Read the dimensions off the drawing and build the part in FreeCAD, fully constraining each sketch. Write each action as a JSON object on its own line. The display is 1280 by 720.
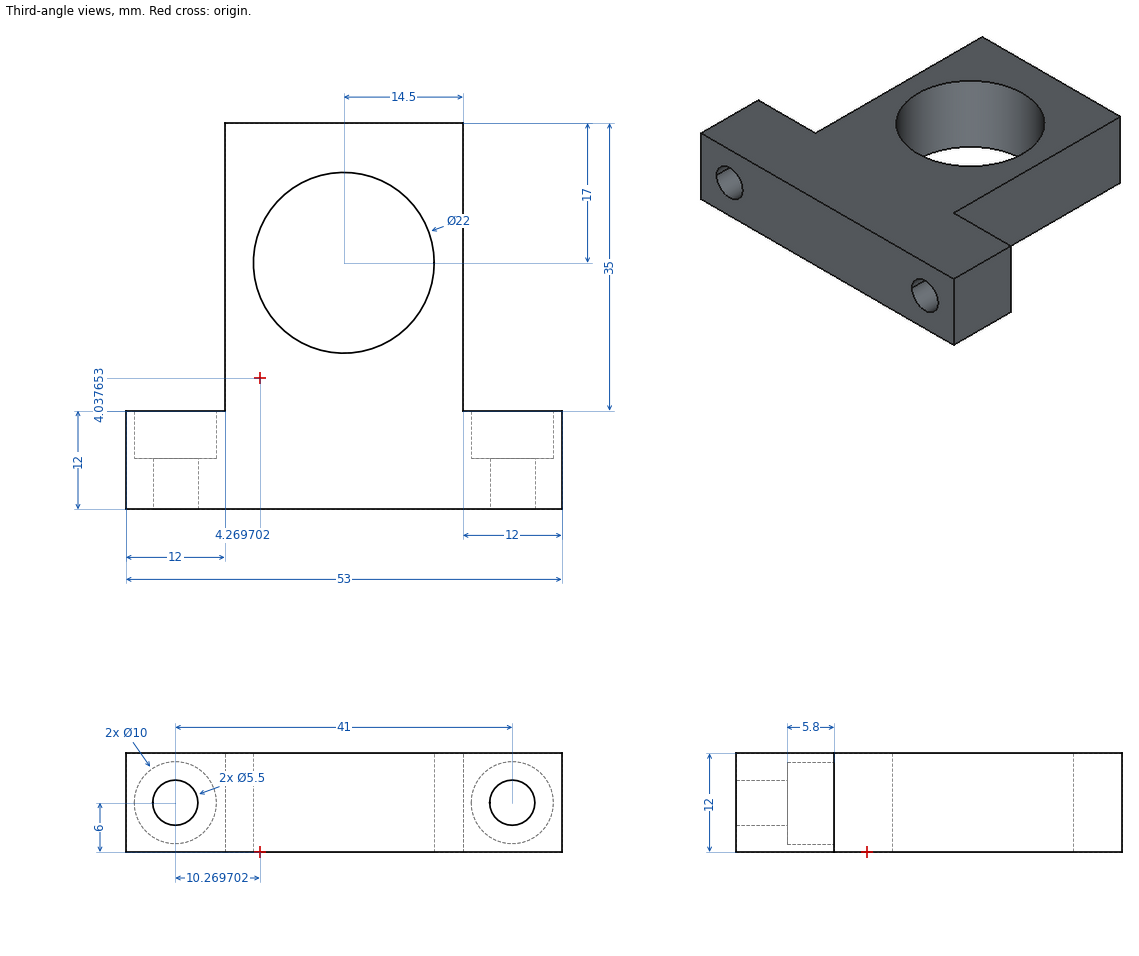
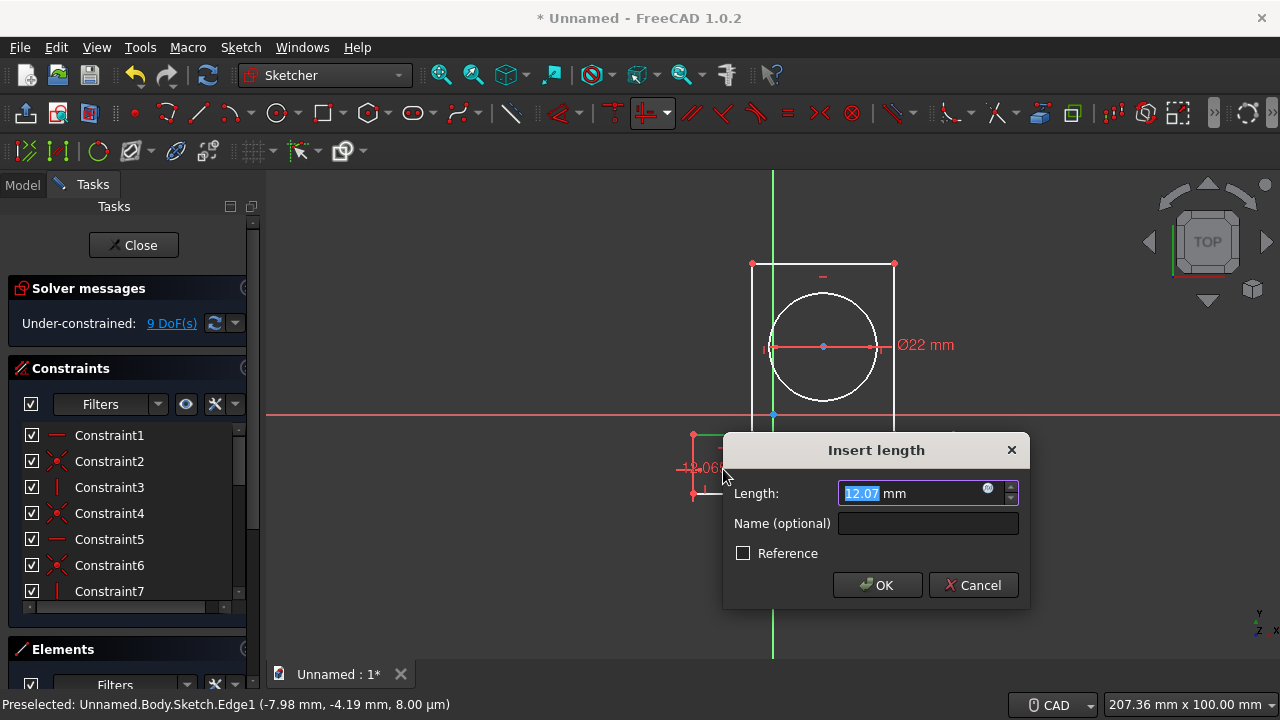
{"action": "type", "text": "12"}
{"action": "key", "text": "Return"}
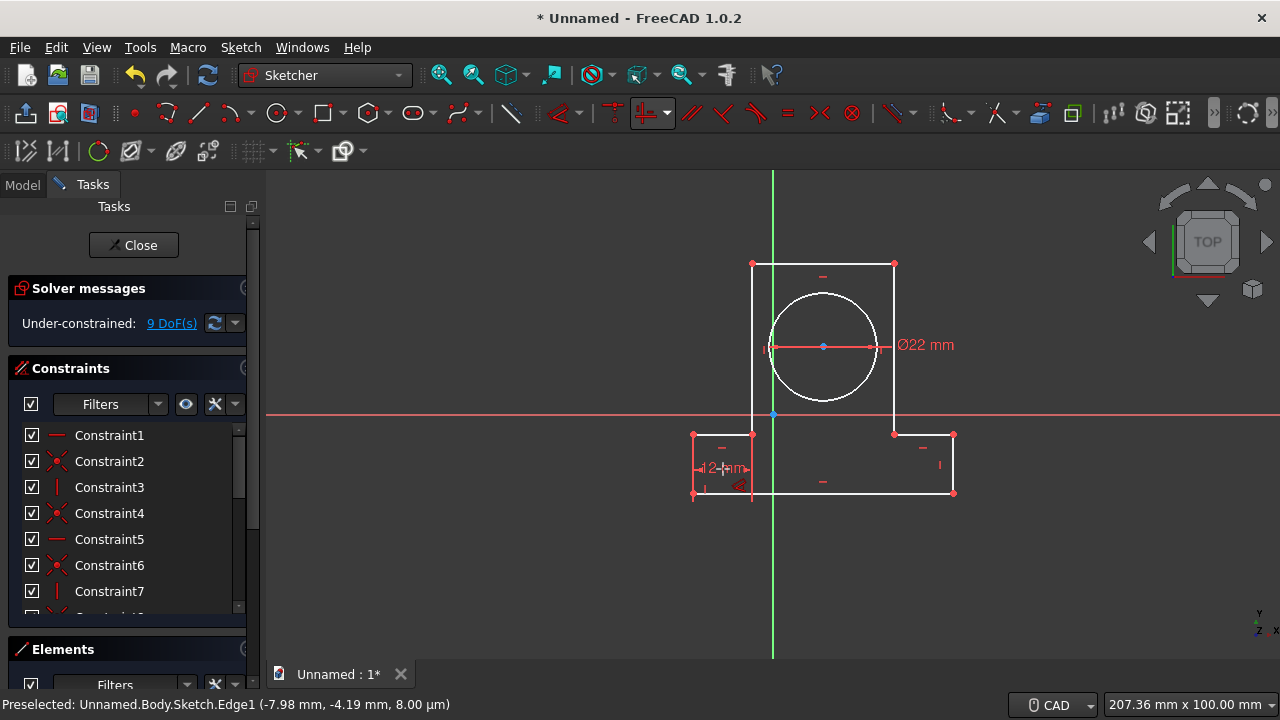
{"action": "left_click", "coordinate": [693, 453]}
{"action": "left_click", "coordinate": [659, 444]}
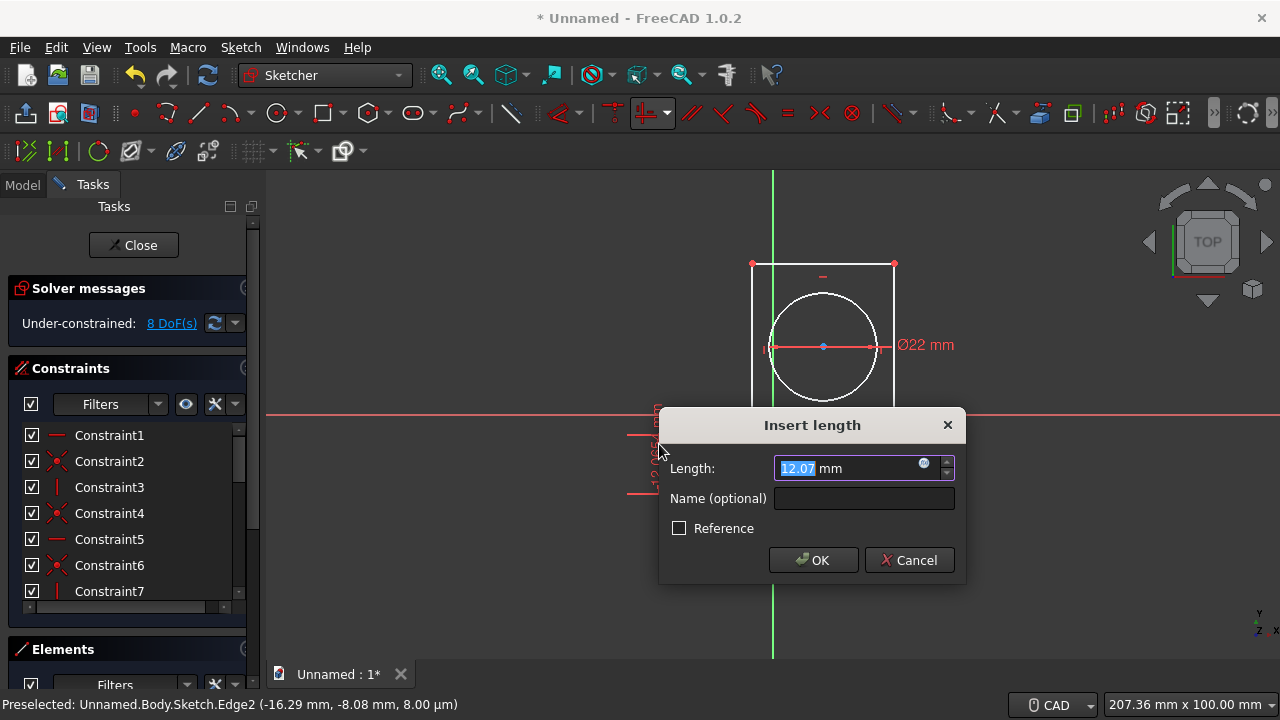
{"action": "type", "text": "12"}
{"action": "key", "text": "Return"}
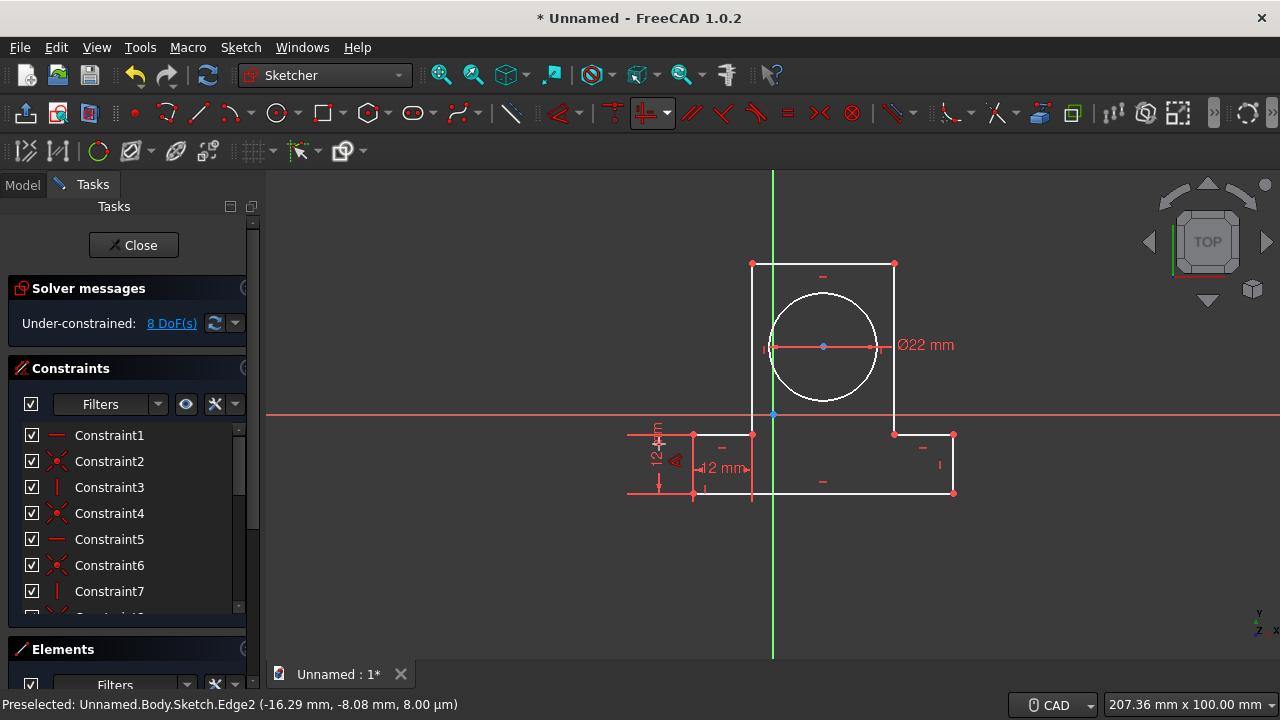
{"action": "left_click", "coordinate": [771, 494]}
{"action": "left_click", "coordinate": [823, 528]}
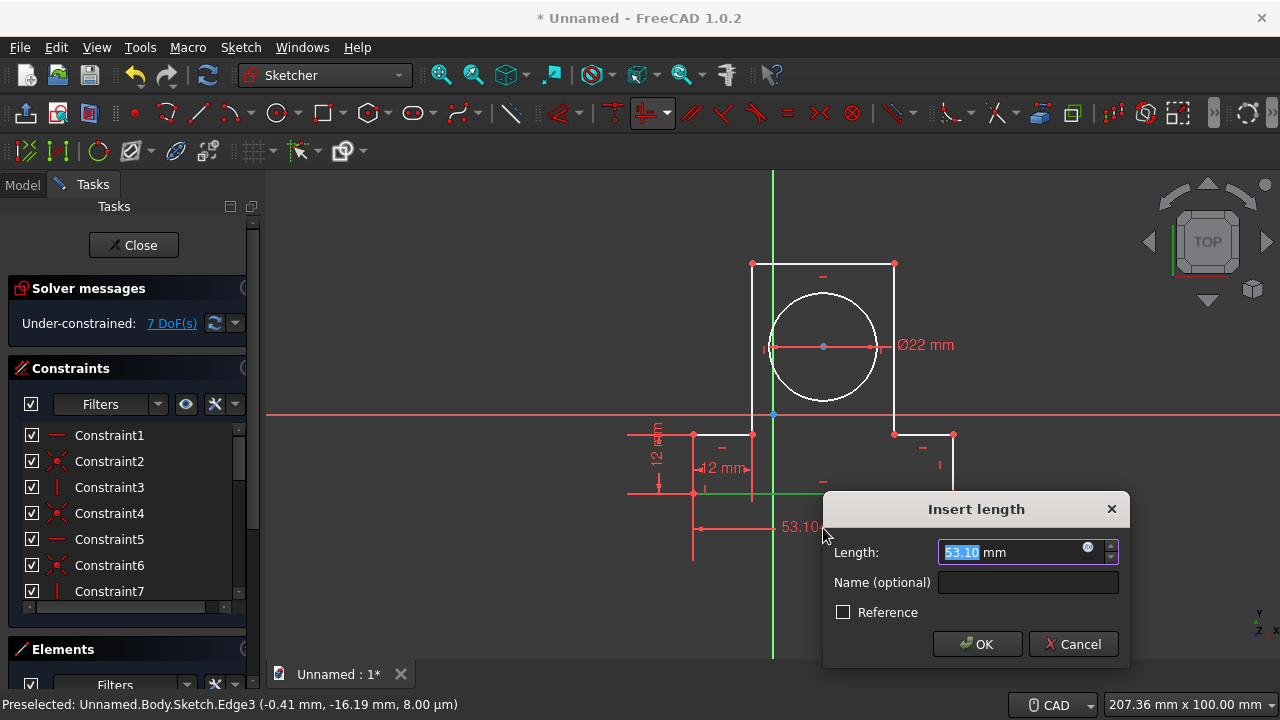
{"action": "type", "text": "53"}
{"action": "key", "text": "Return"}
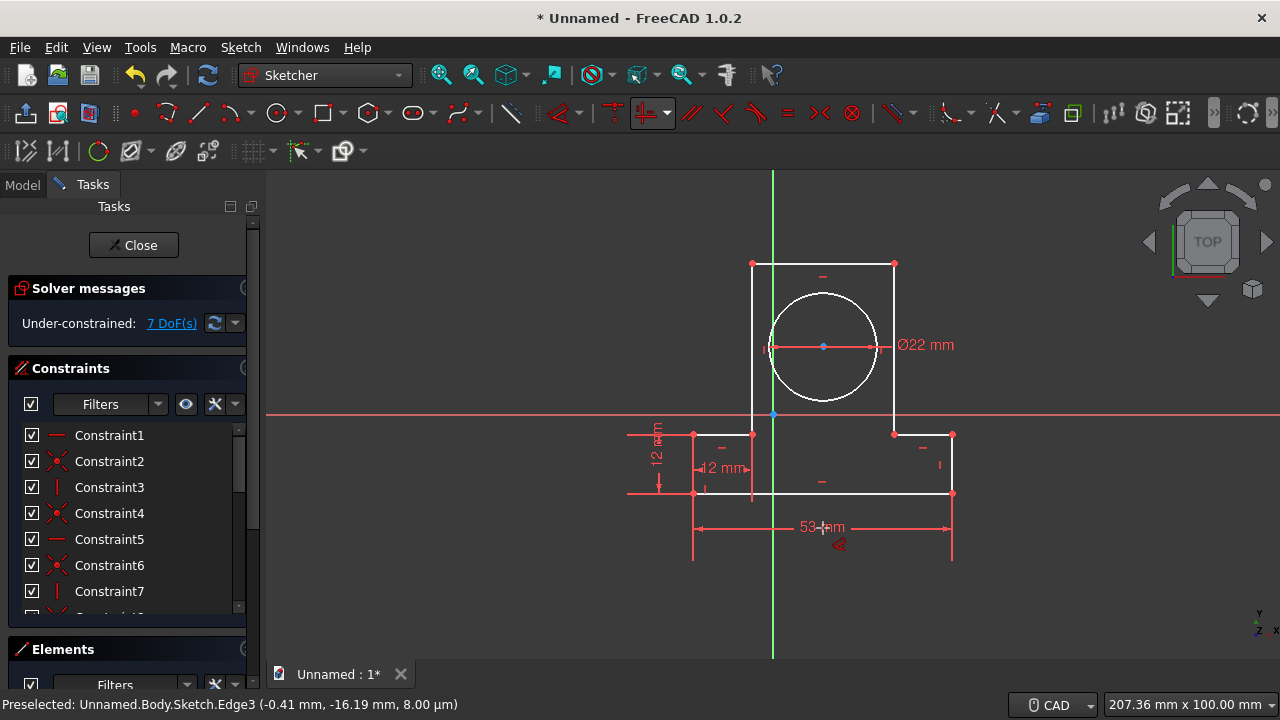
{"action": "left_click", "coordinate": [952, 476]}
{"action": "left_click", "coordinate": [986, 464]}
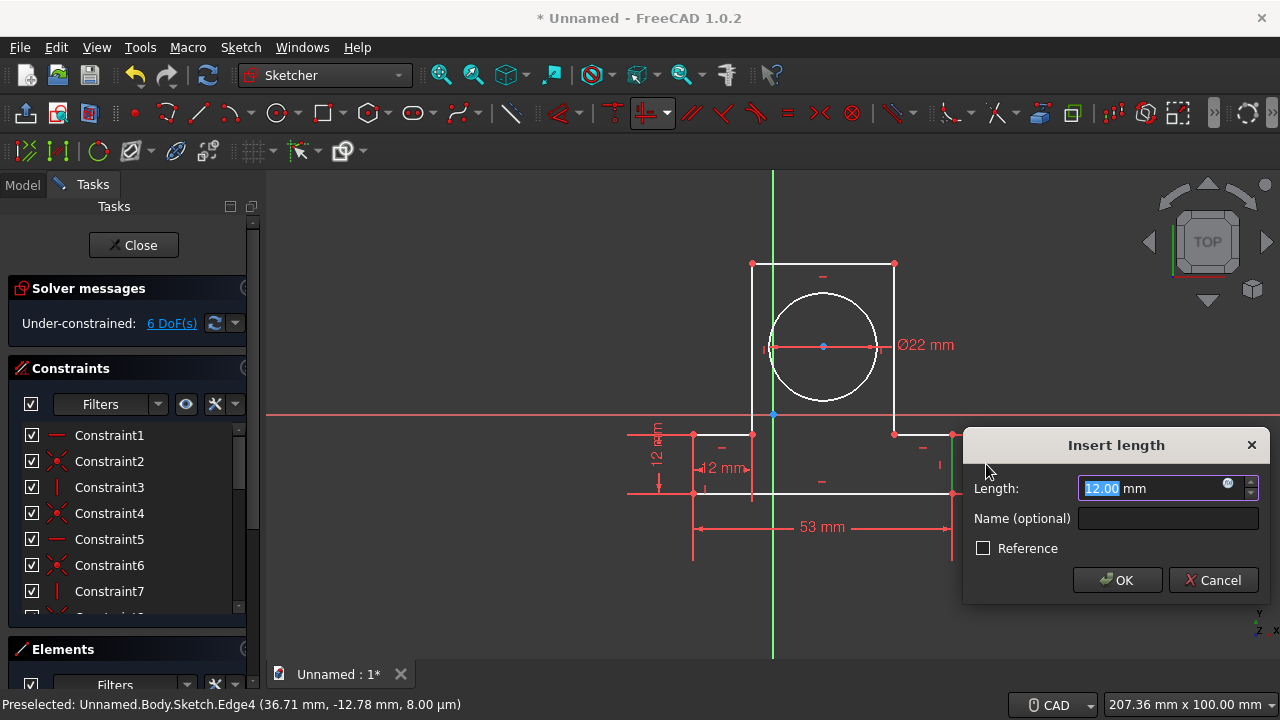
{"action": "type", "text": "12"}
{"action": "key", "text": "Return"}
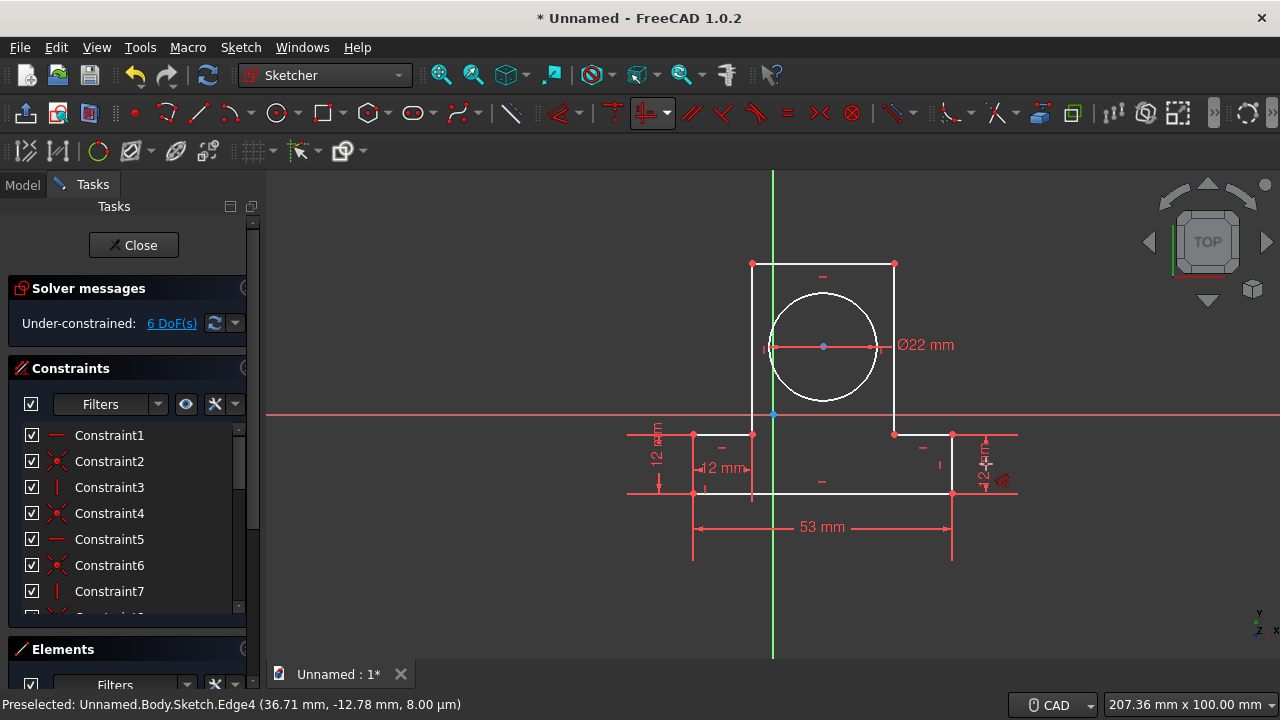
{"action": "left_click", "coordinate": [935, 435]}
{"action": "left_click", "coordinate": [910, 469]}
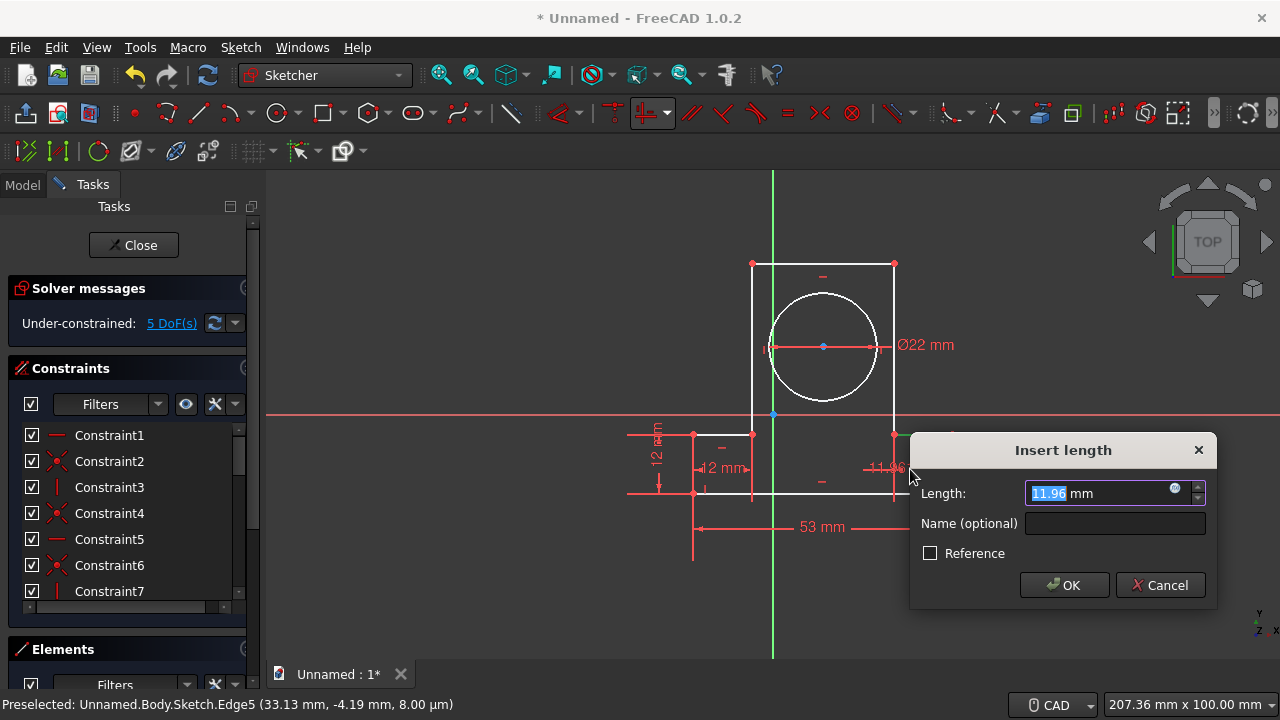
{"action": "type", "text": "12"}
{"action": "key", "text": "Return"}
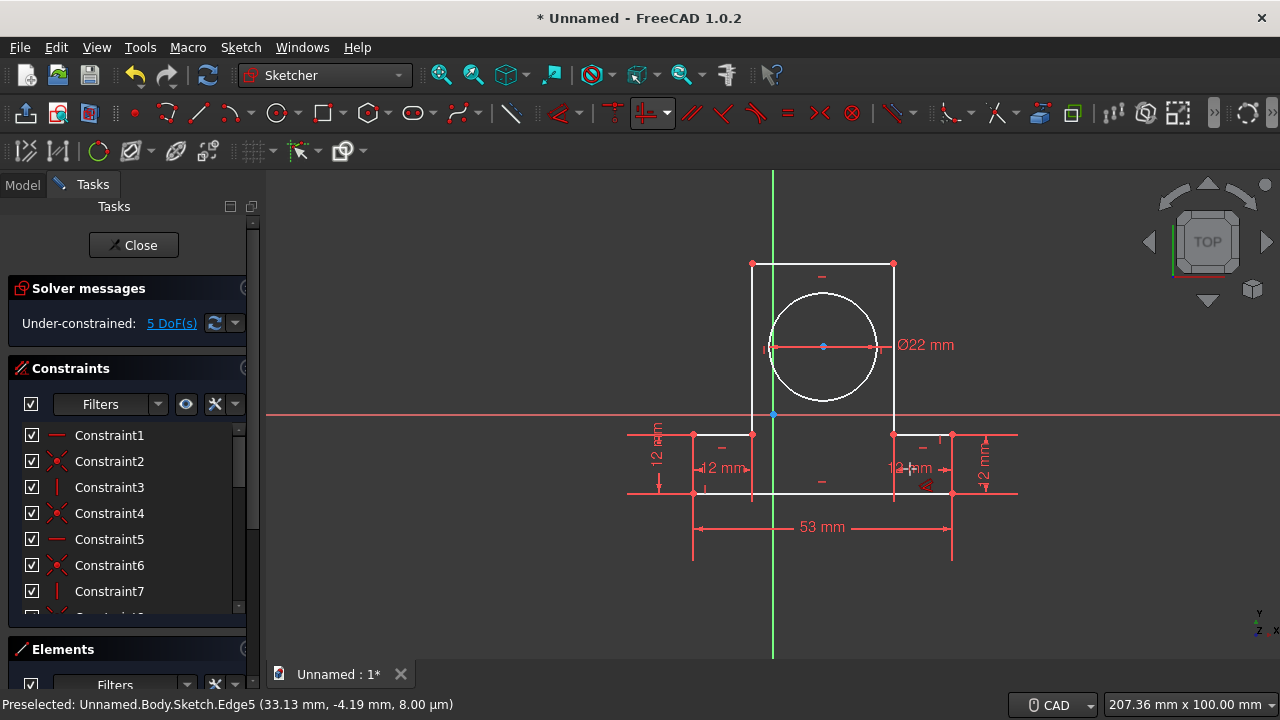
{"action": "left_click", "coordinate": [894, 384]}
{"action": "left_click", "coordinate": [928, 350]}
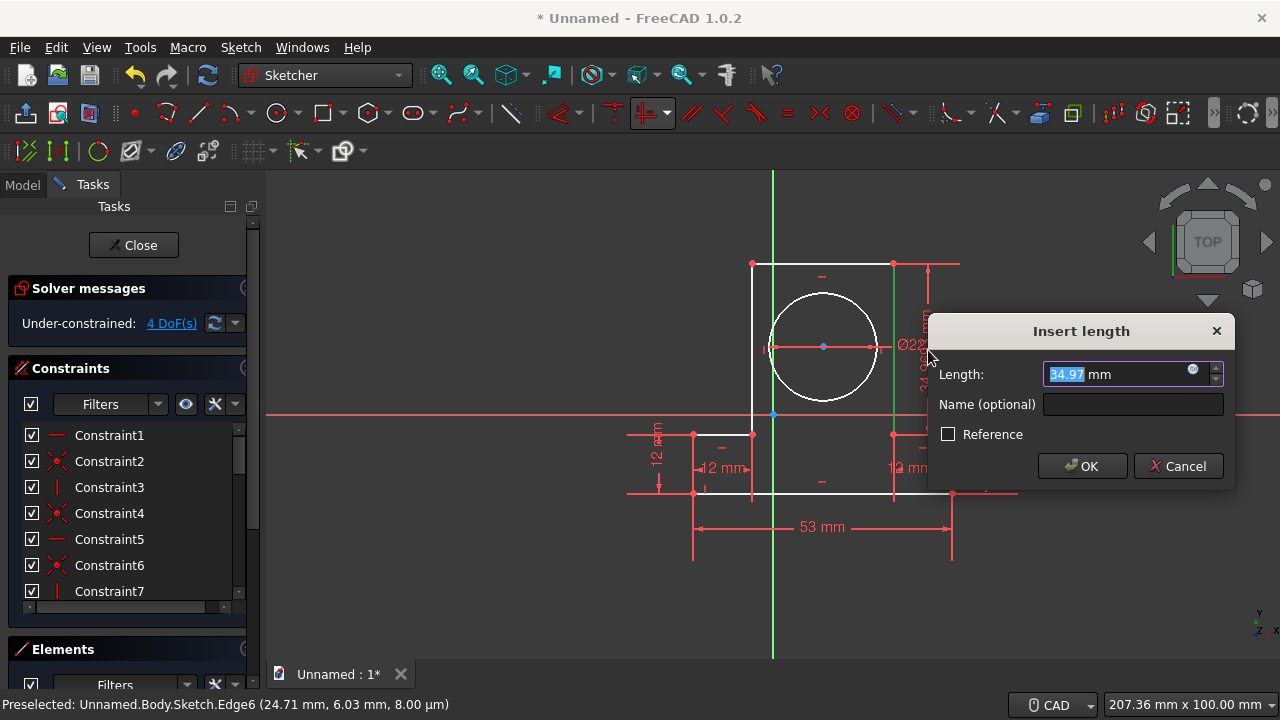
{"action": "type", "text": "35"}
{"action": "key", "text": "Return"}